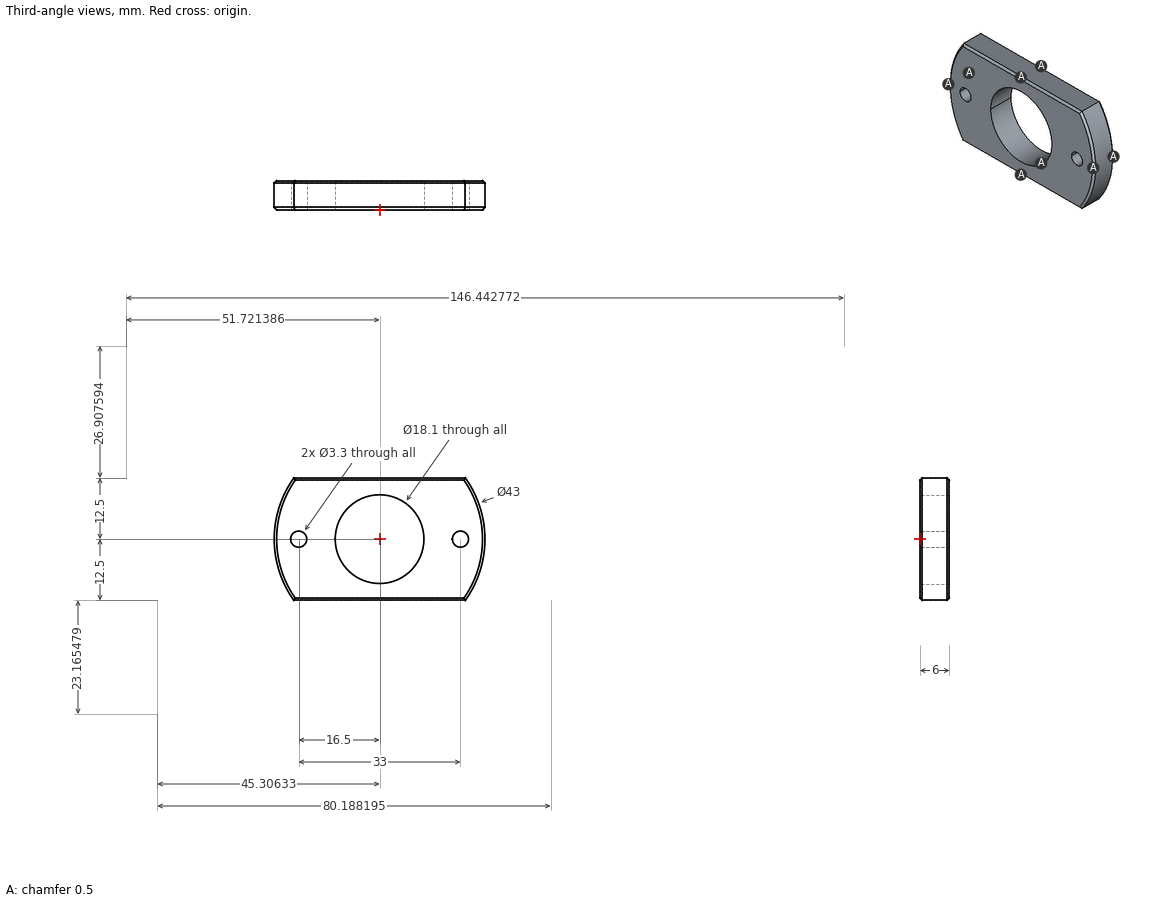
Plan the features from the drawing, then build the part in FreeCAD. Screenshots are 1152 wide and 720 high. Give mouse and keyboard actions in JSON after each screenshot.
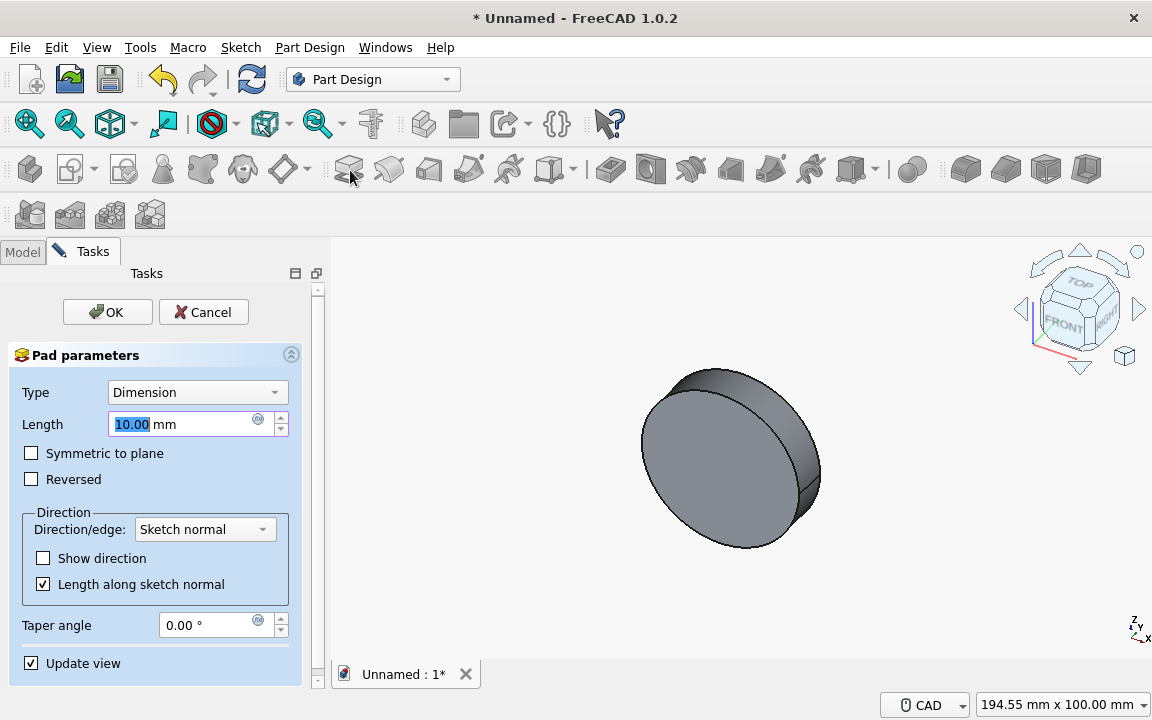
{"action": "type", "text": "6"}
{"action": "key", "text": "Tab"}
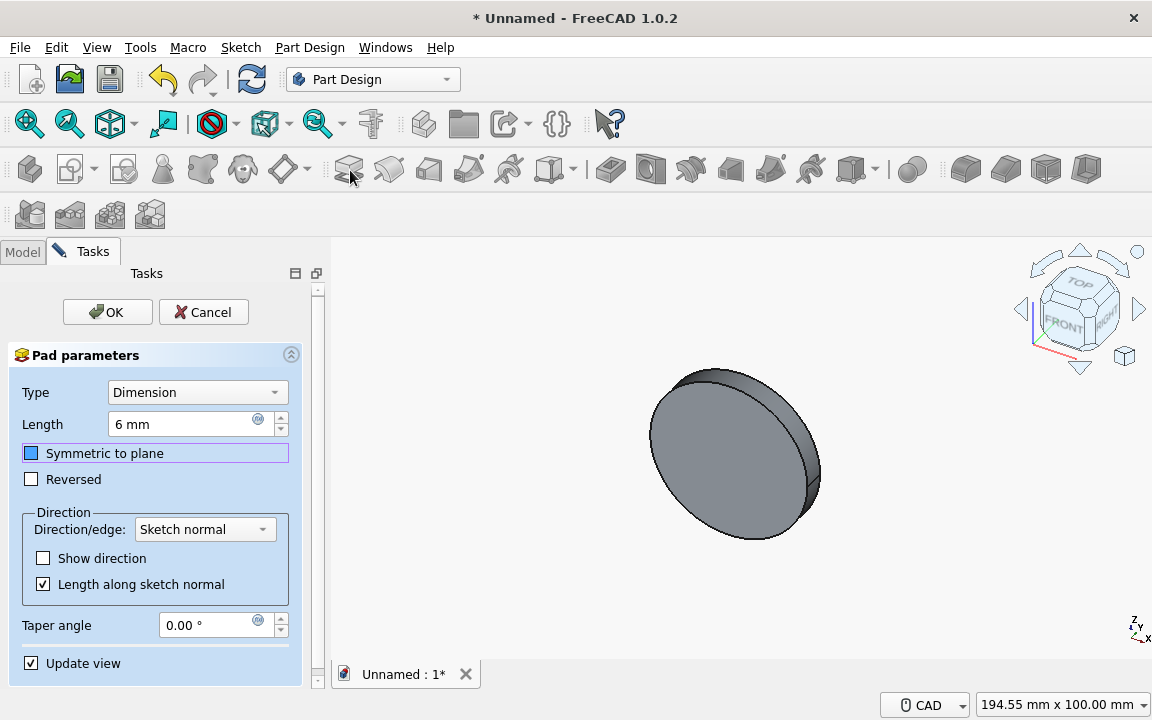
{"action": "left_click", "coordinate": [30, 479]}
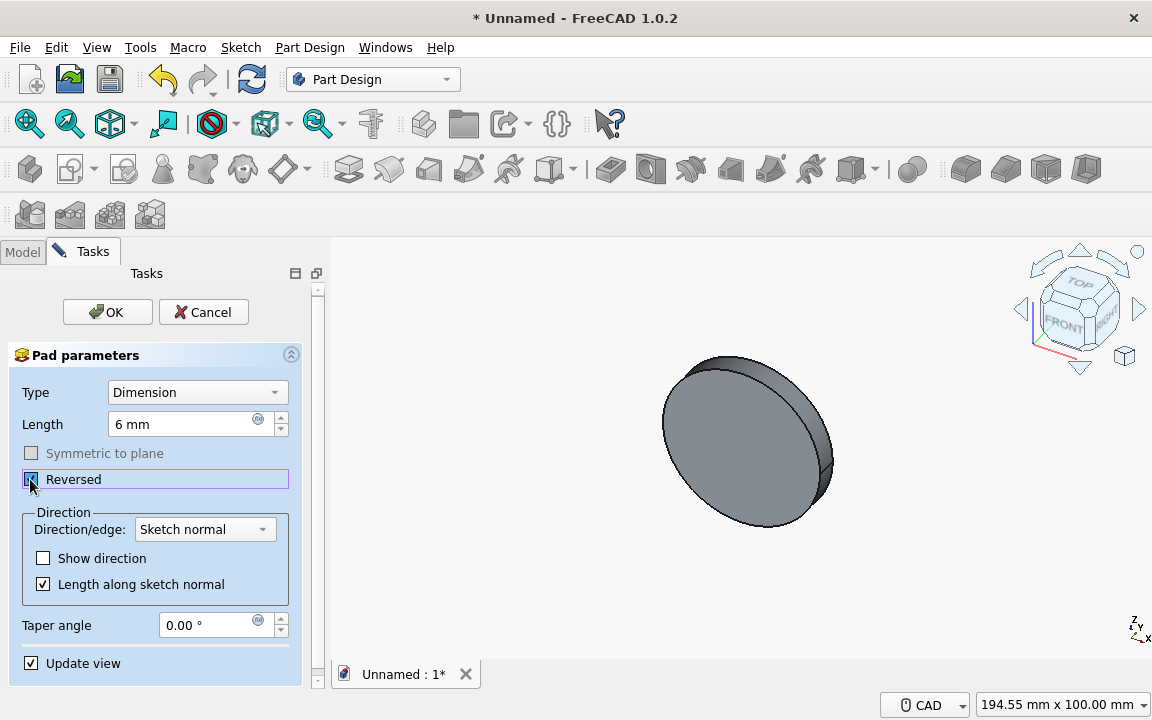
{"action": "left_click", "coordinate": [108, 312]}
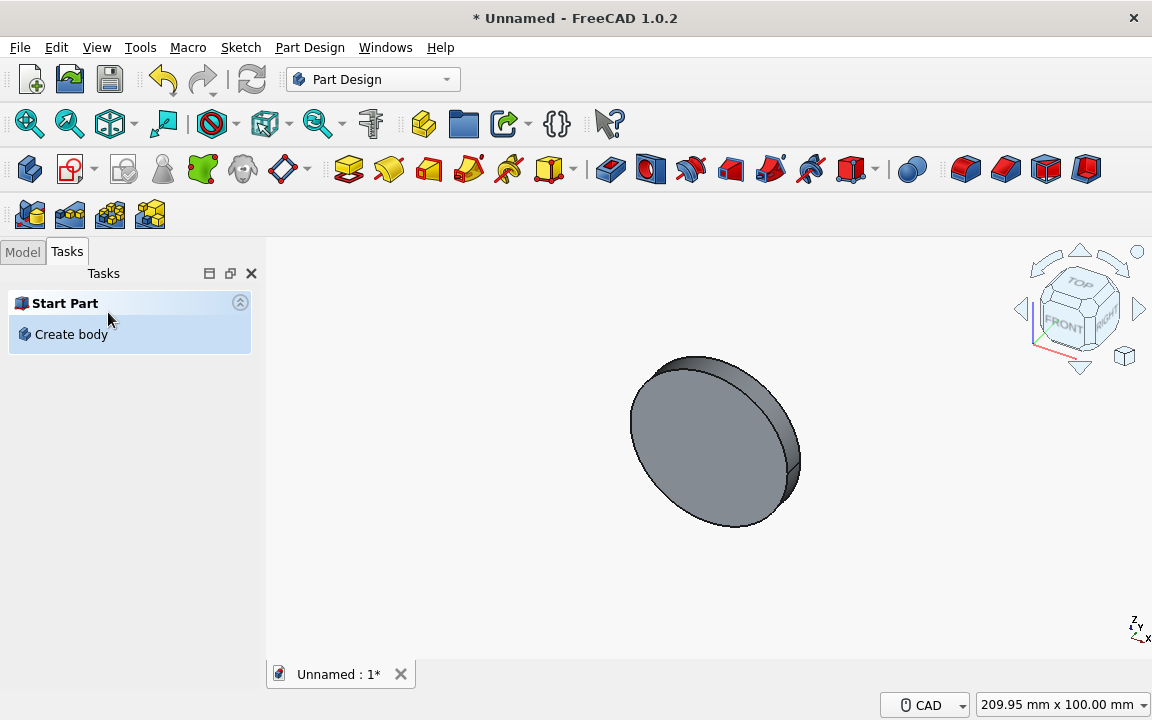
{"action": "key", "text": "4"}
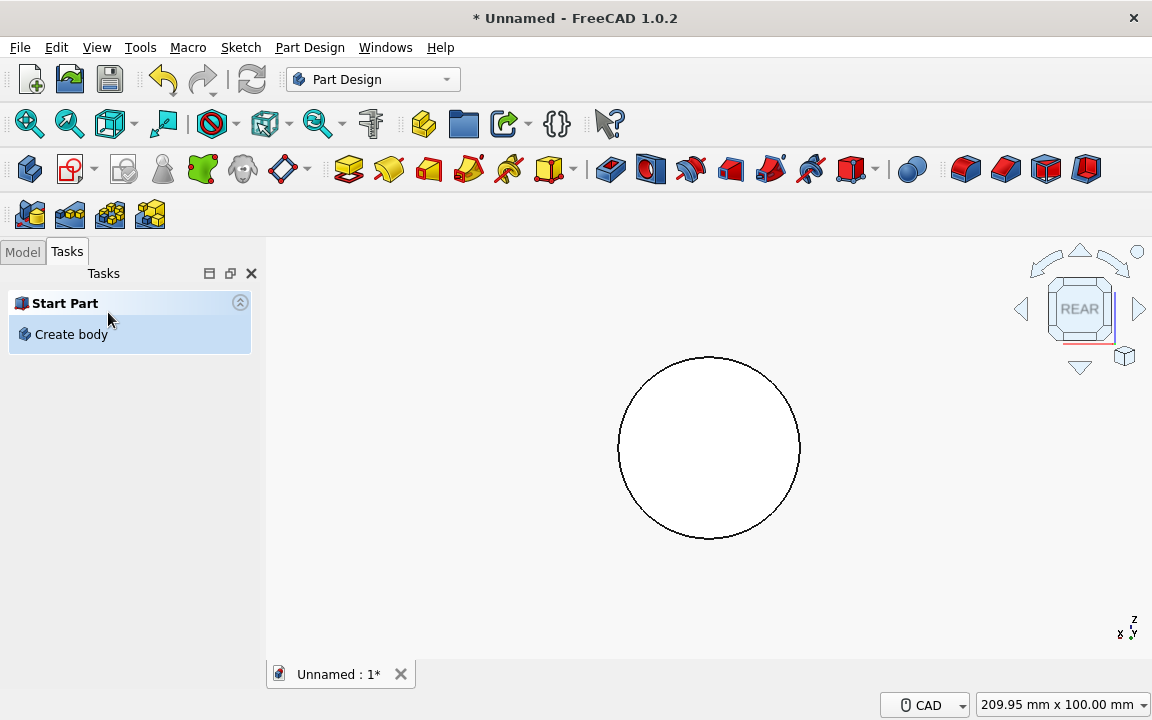
{"action": "left_click", "coordinate": [30, 124]}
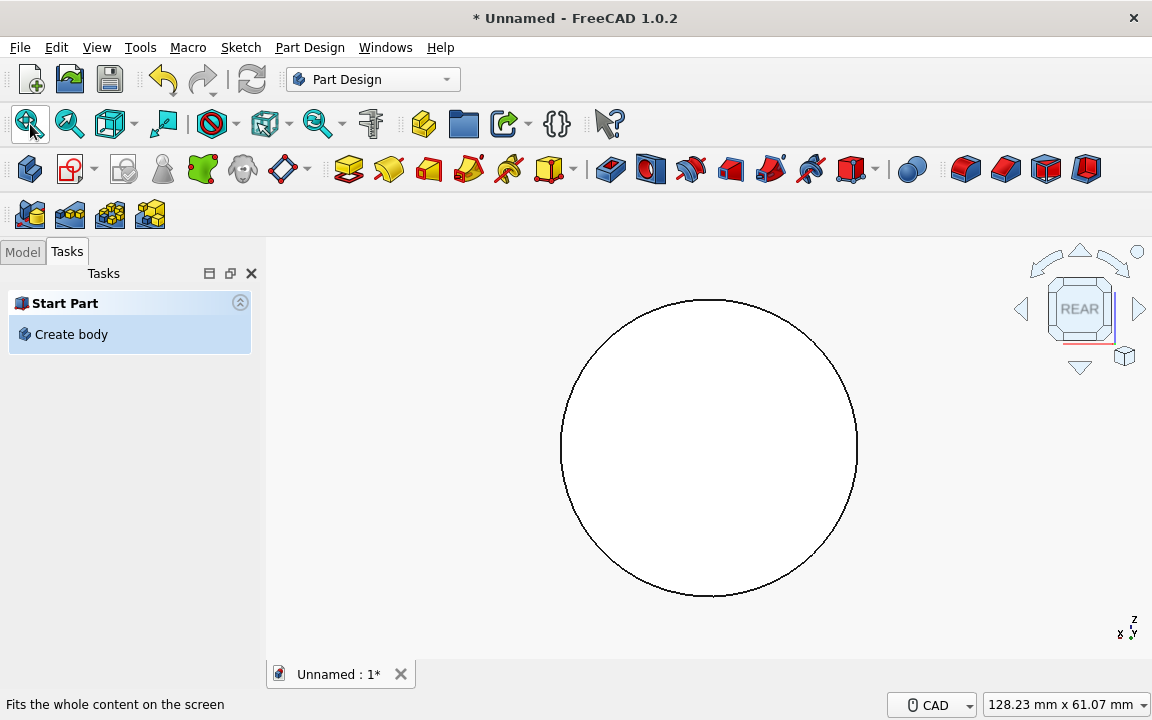
{"action": "left_click", "coordinate": [709, 447]}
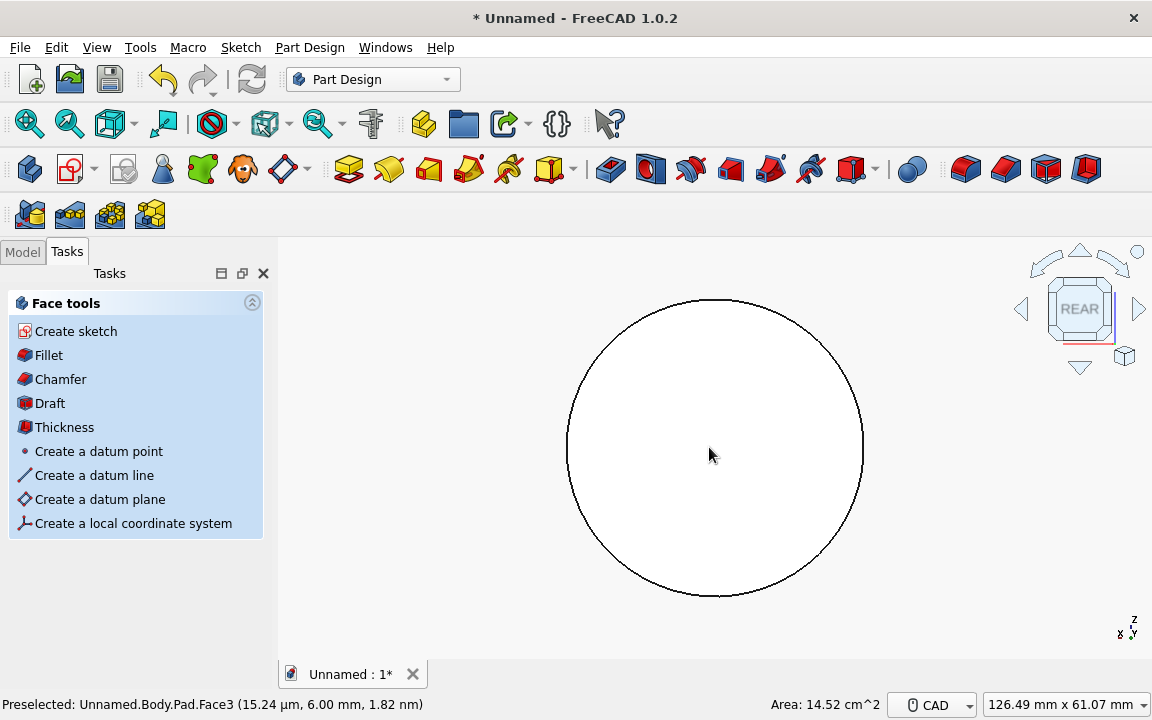
{"action": "left_click", "coordinate": [70, 170]}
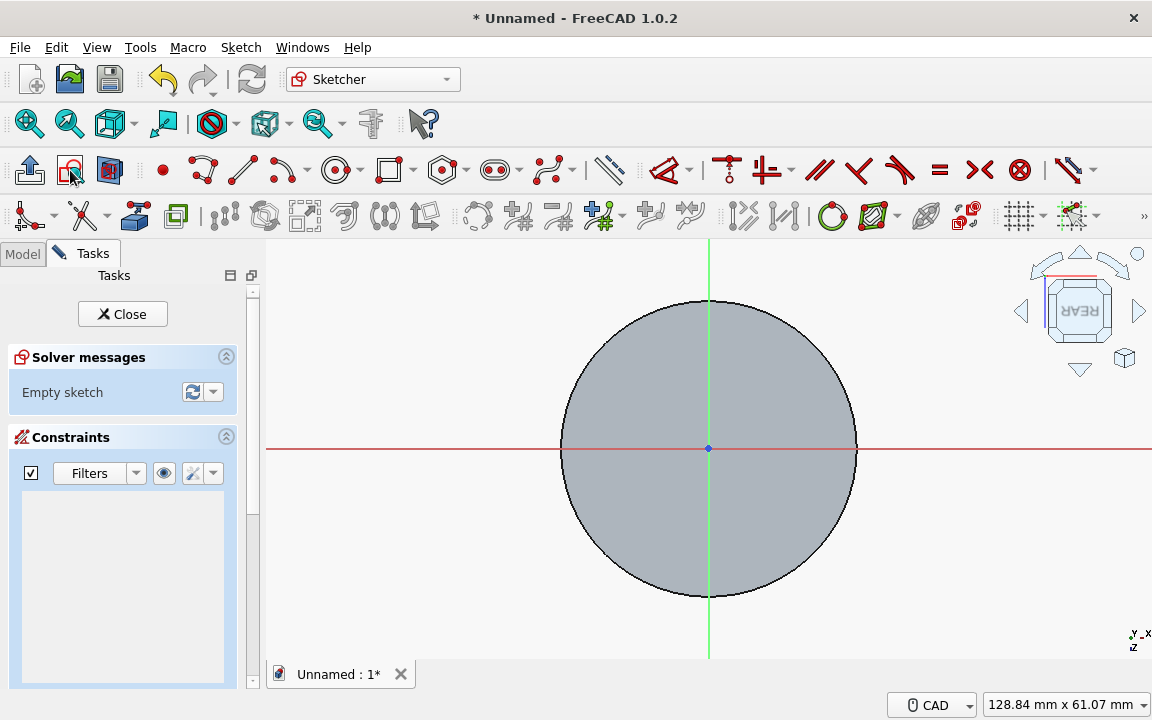
{"action": "scroll", "coordinate": [792, 449], "scroll_direction": "up", "scroll_amount": 3}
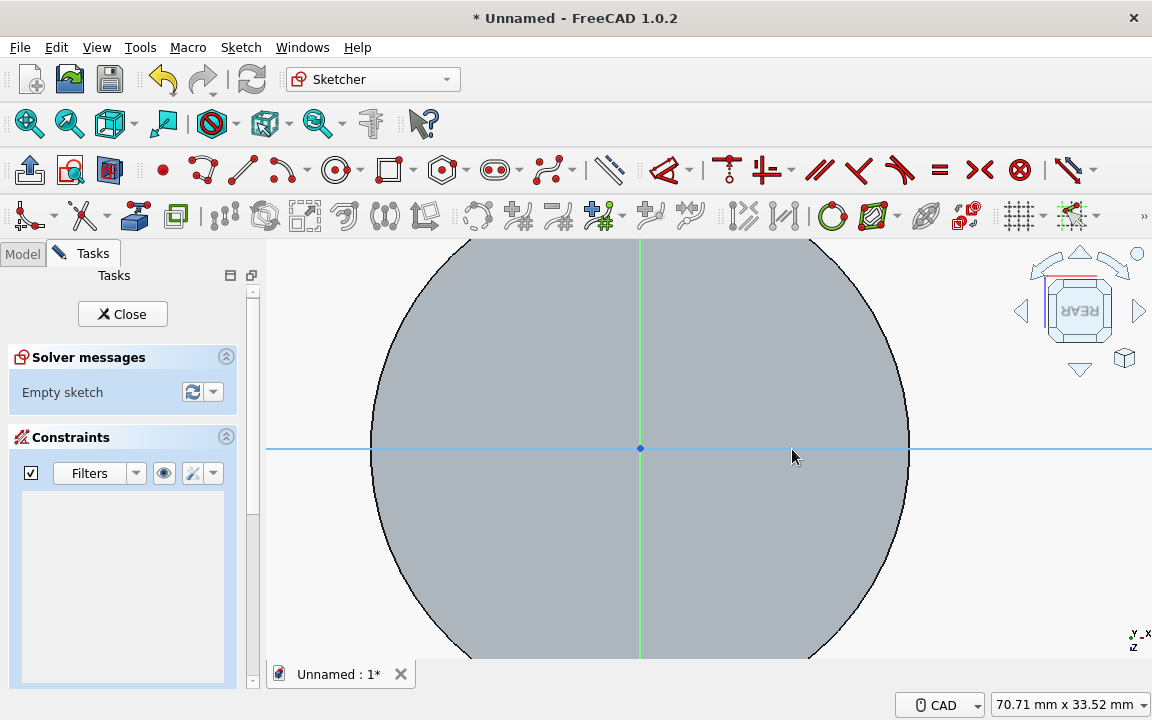
{"action": "left_click", "coordinate": [336, 170]}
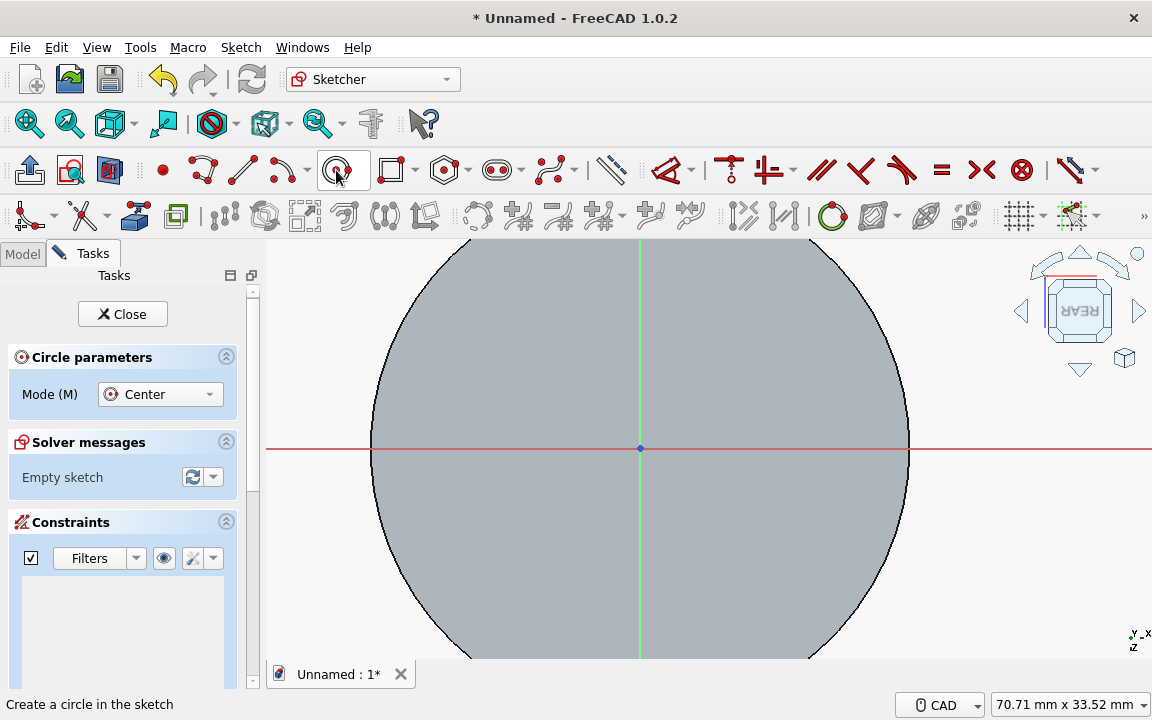
{"action": "left_click", "coordinate": [433, 449]}
{"action": "left_click", "coordinate": [448, 434]}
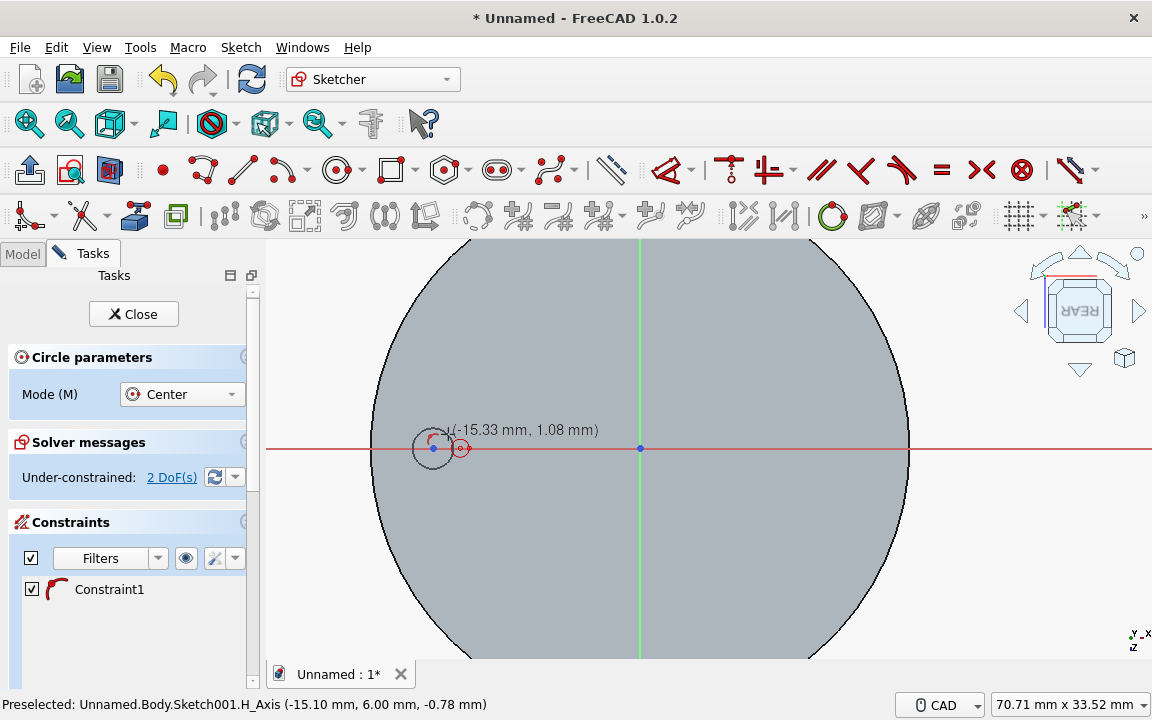
{"action": "left_click", "coordinate": [847, 449]}
{"action": "left_click", "coordinate": [861, 434]}
{"action": "key", "text": "Escape"}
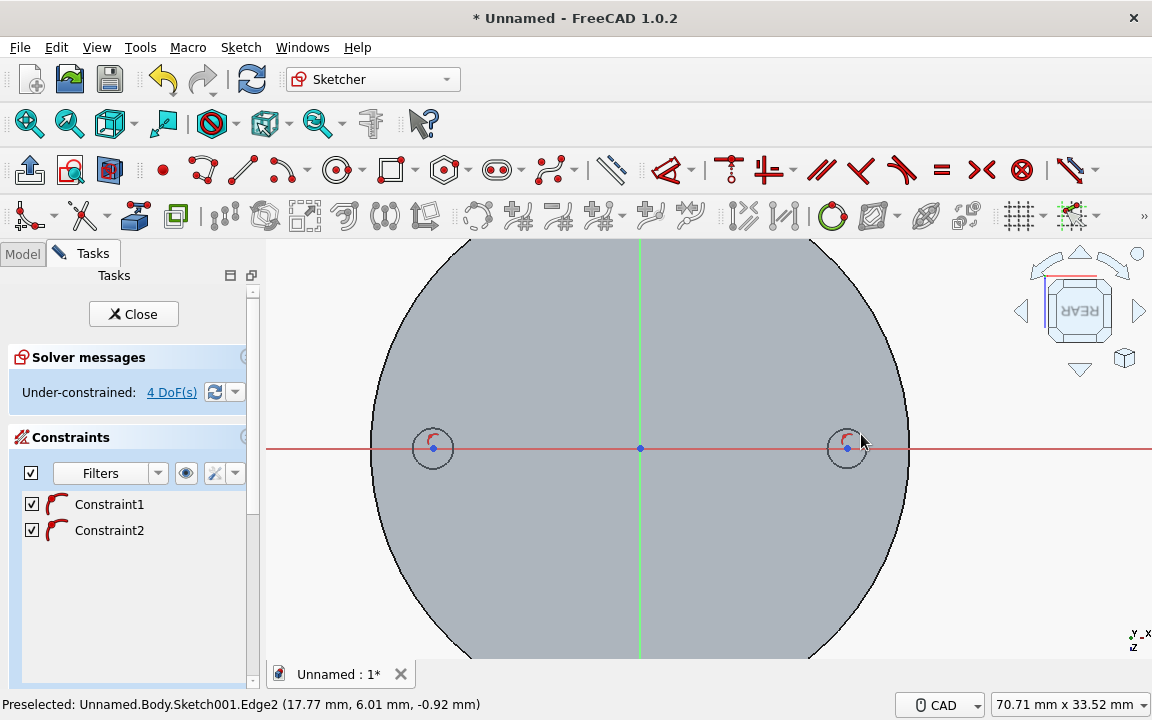
{"action": "left_click", "coordinate": [447, 434]}